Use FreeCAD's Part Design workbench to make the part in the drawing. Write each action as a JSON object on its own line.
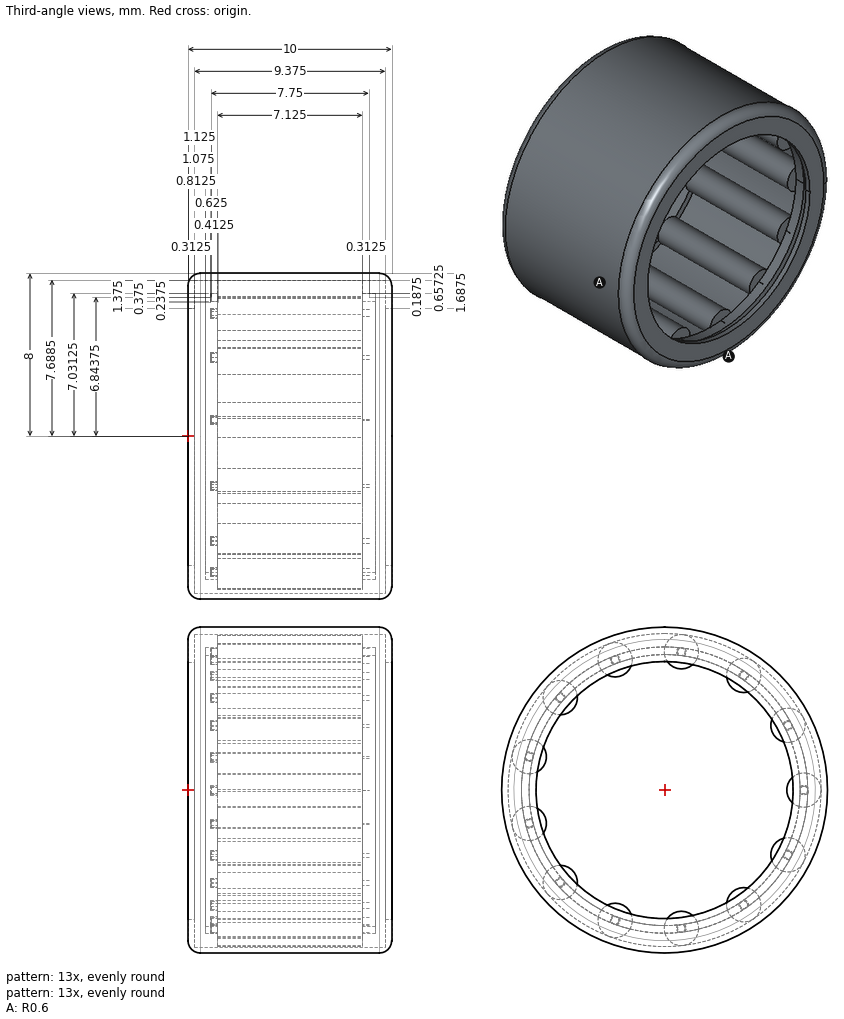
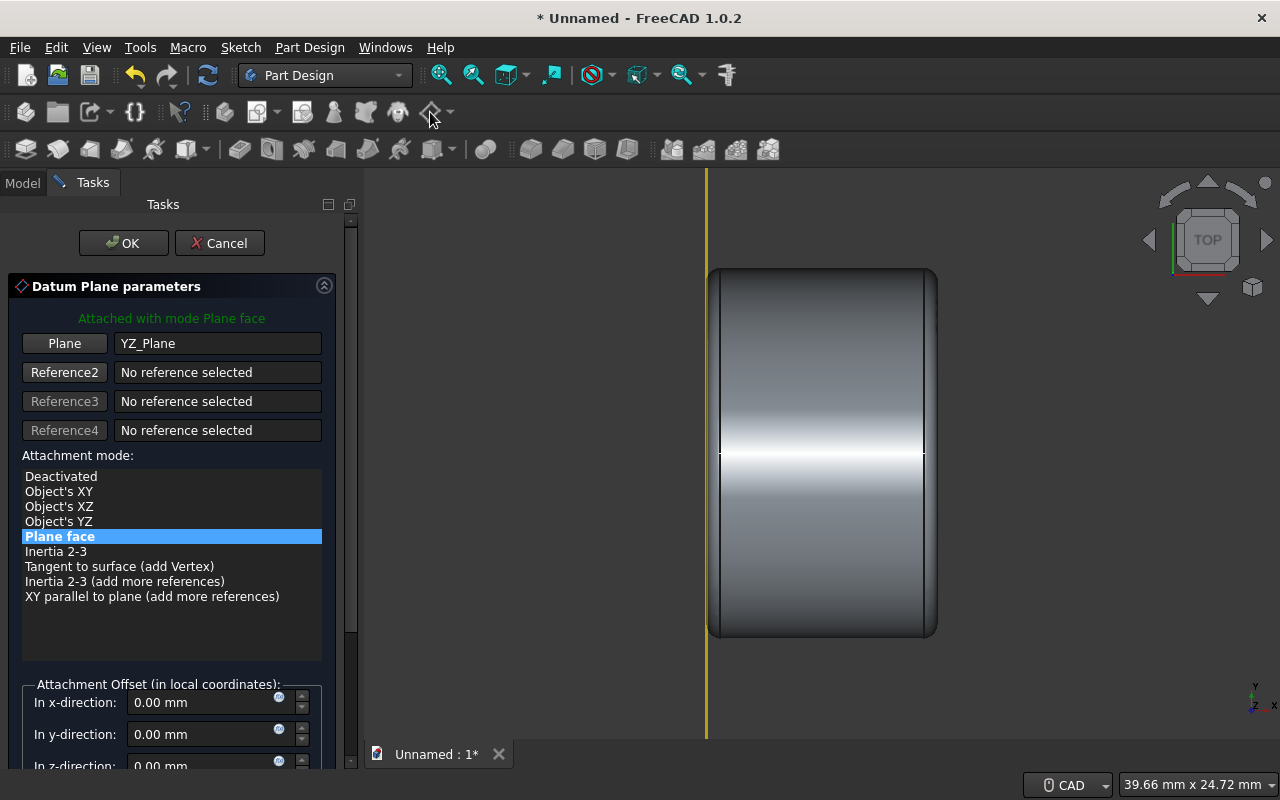
{"action": "scroll", "coordinate": [351, 491], "scroll_direction": "down", "scroll_amount": 2}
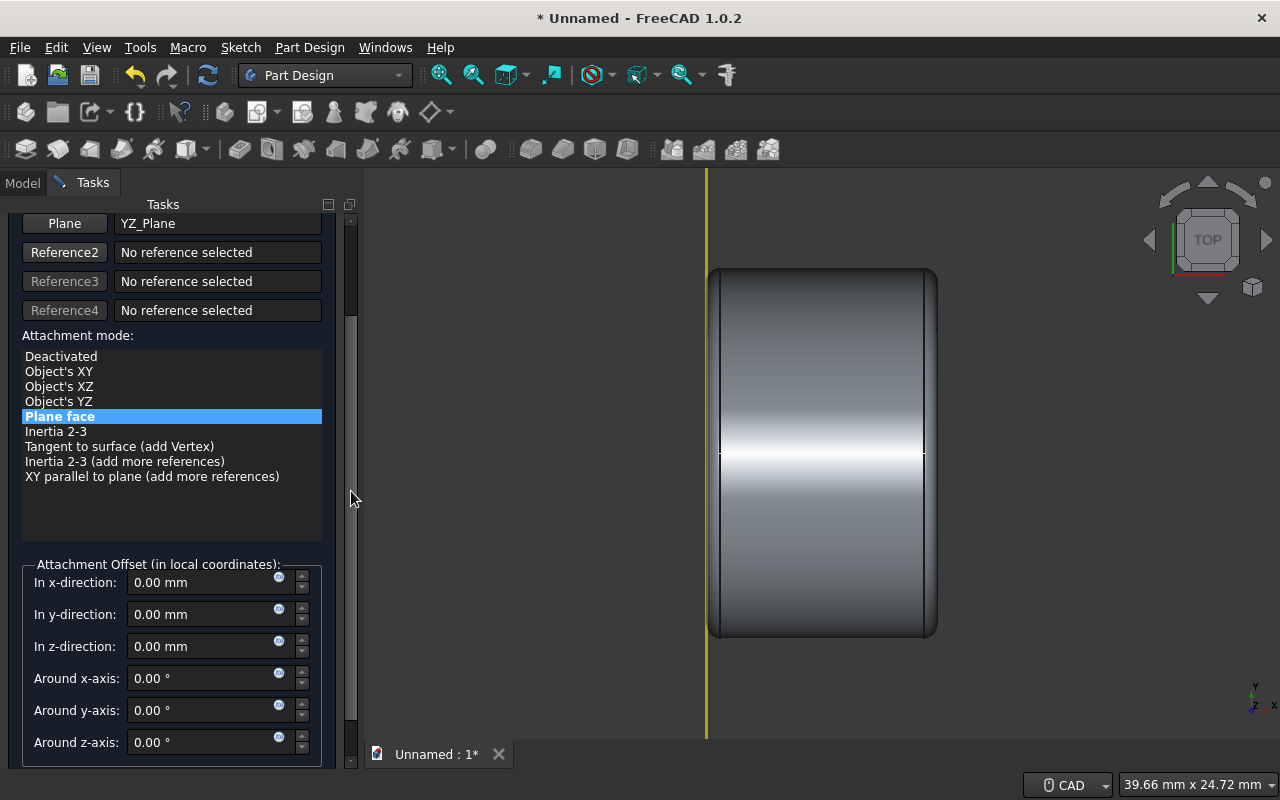
{"action": "triple_click", "coordinate": [210, 646]}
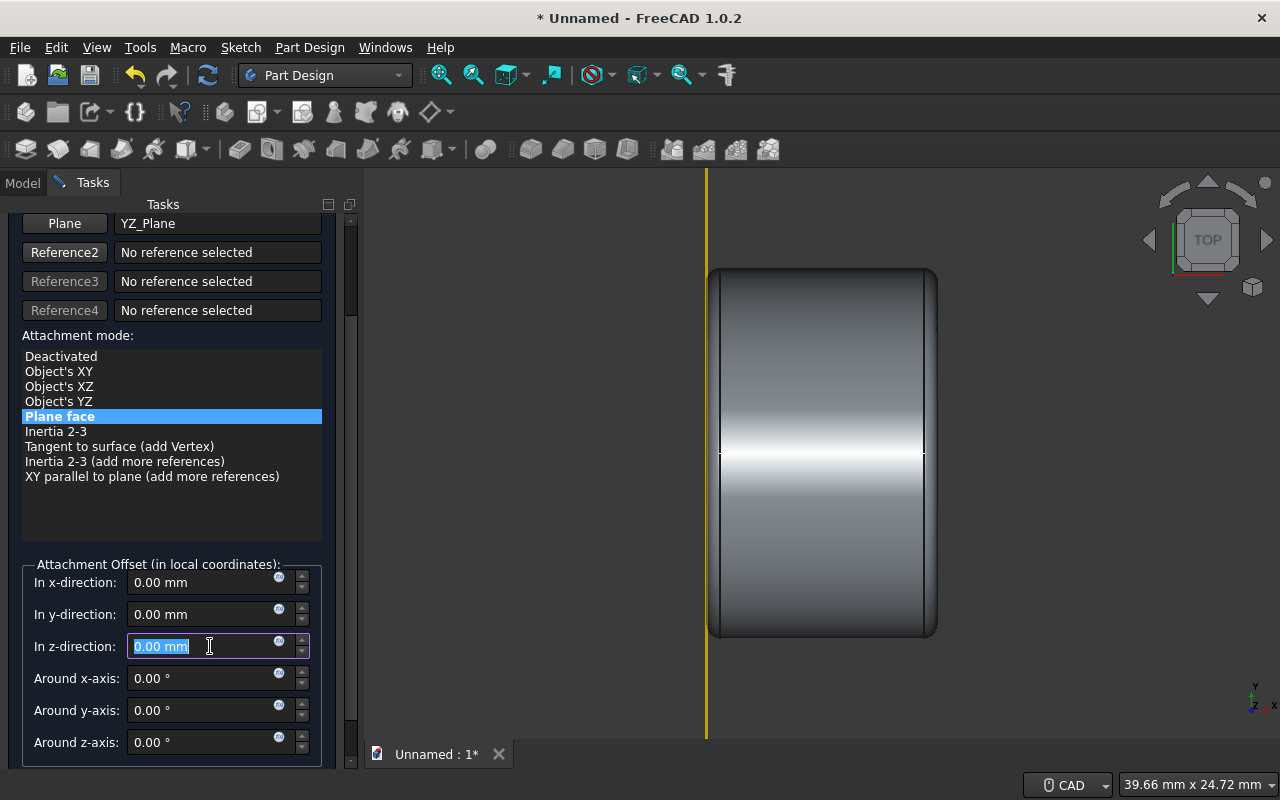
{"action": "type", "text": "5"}
{"action": "key", "text": "Tab"}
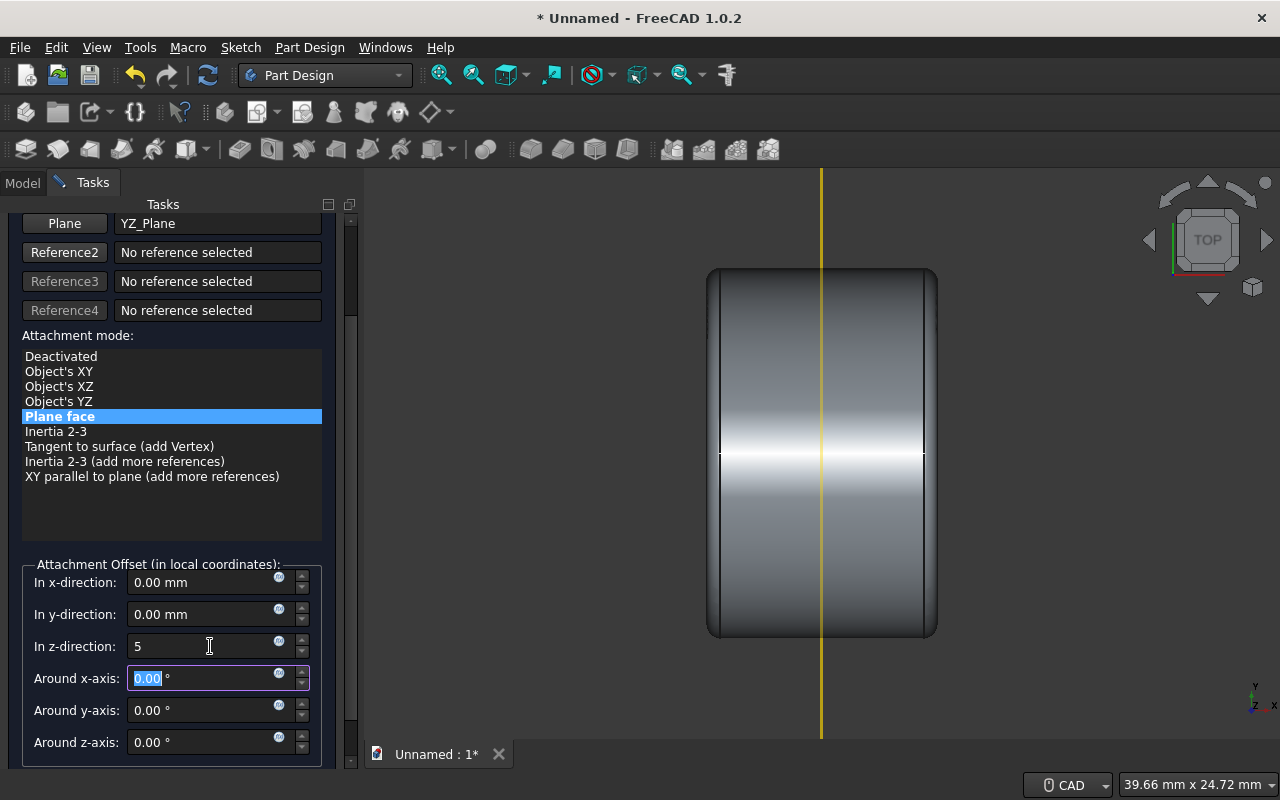
{"action": "scroll", "coordinate": [351, 491], "scroll_direction": "up", "scroll_amount": 3}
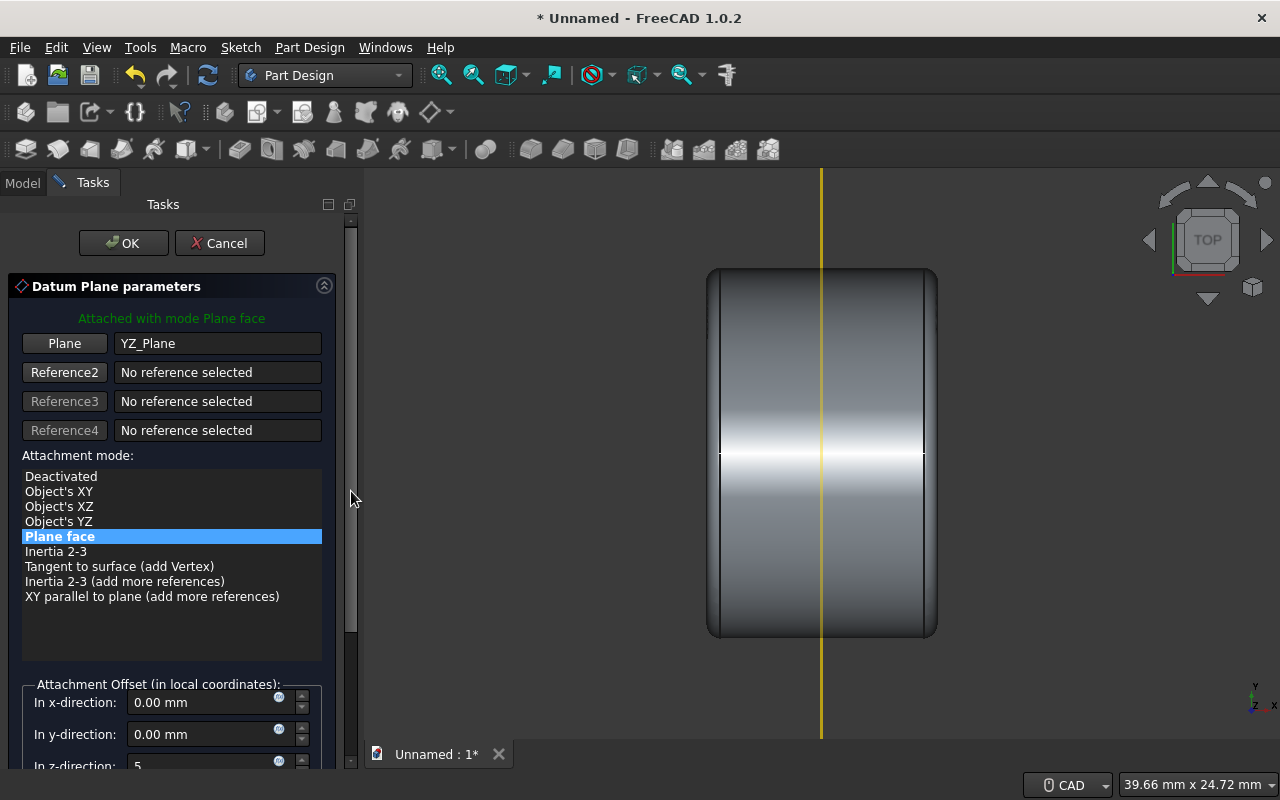
{"action": "left_click", "coordinate": [124, 243]}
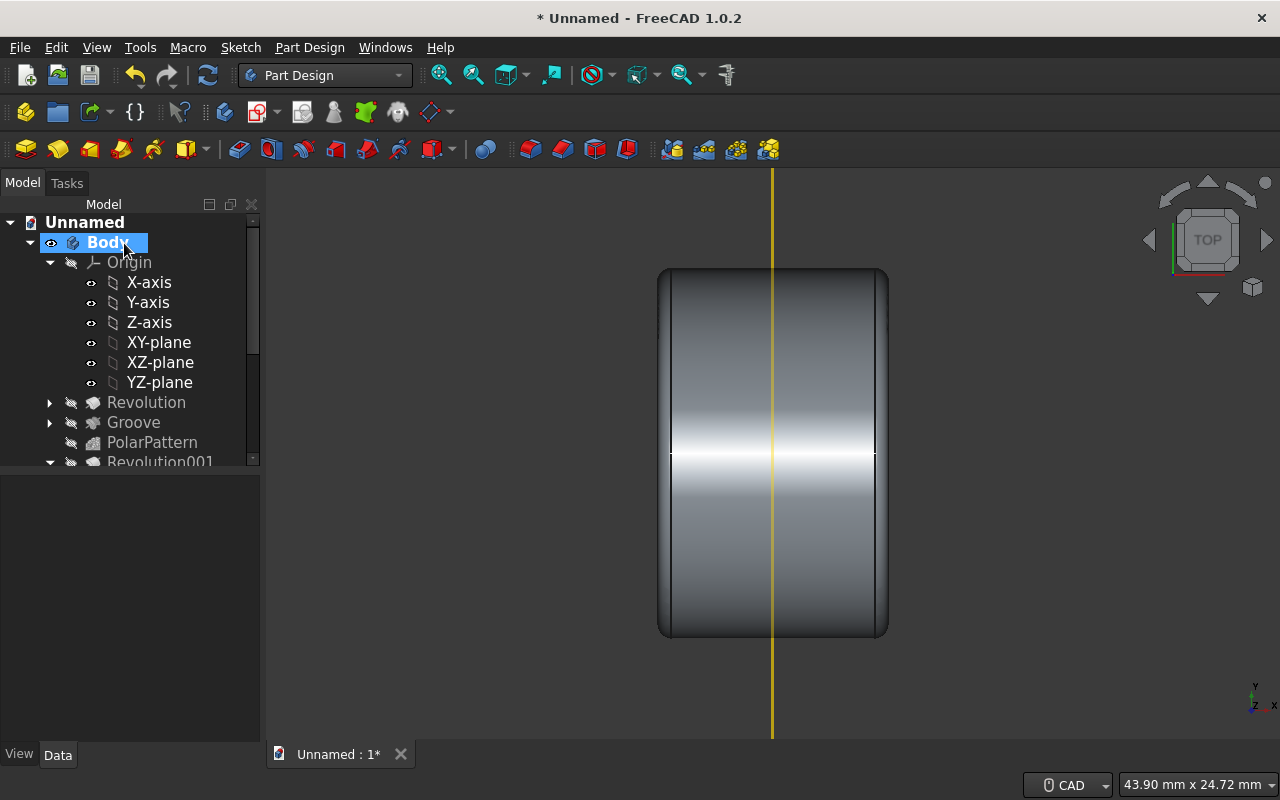
{"action": "left_click", "coordinate": [116, 463]}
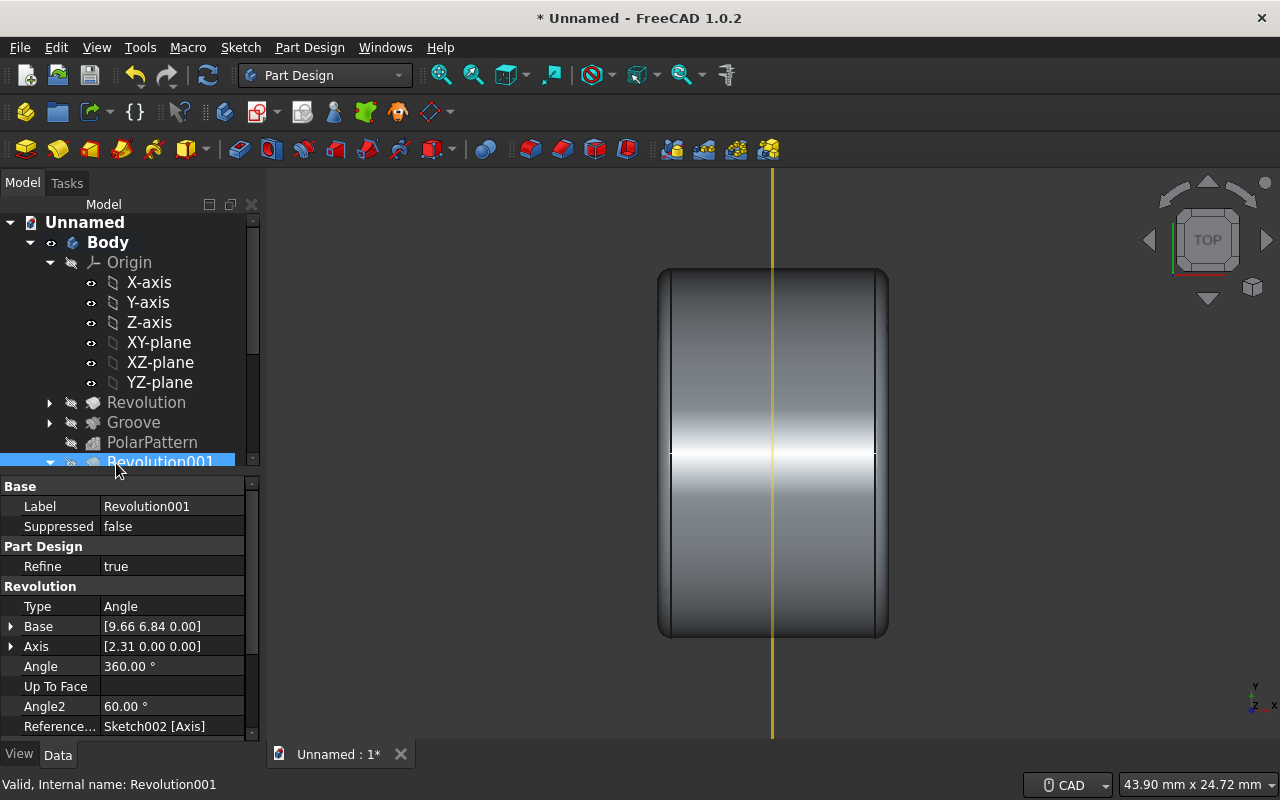
{"action": "left_click", "coordinate": [672, 150]}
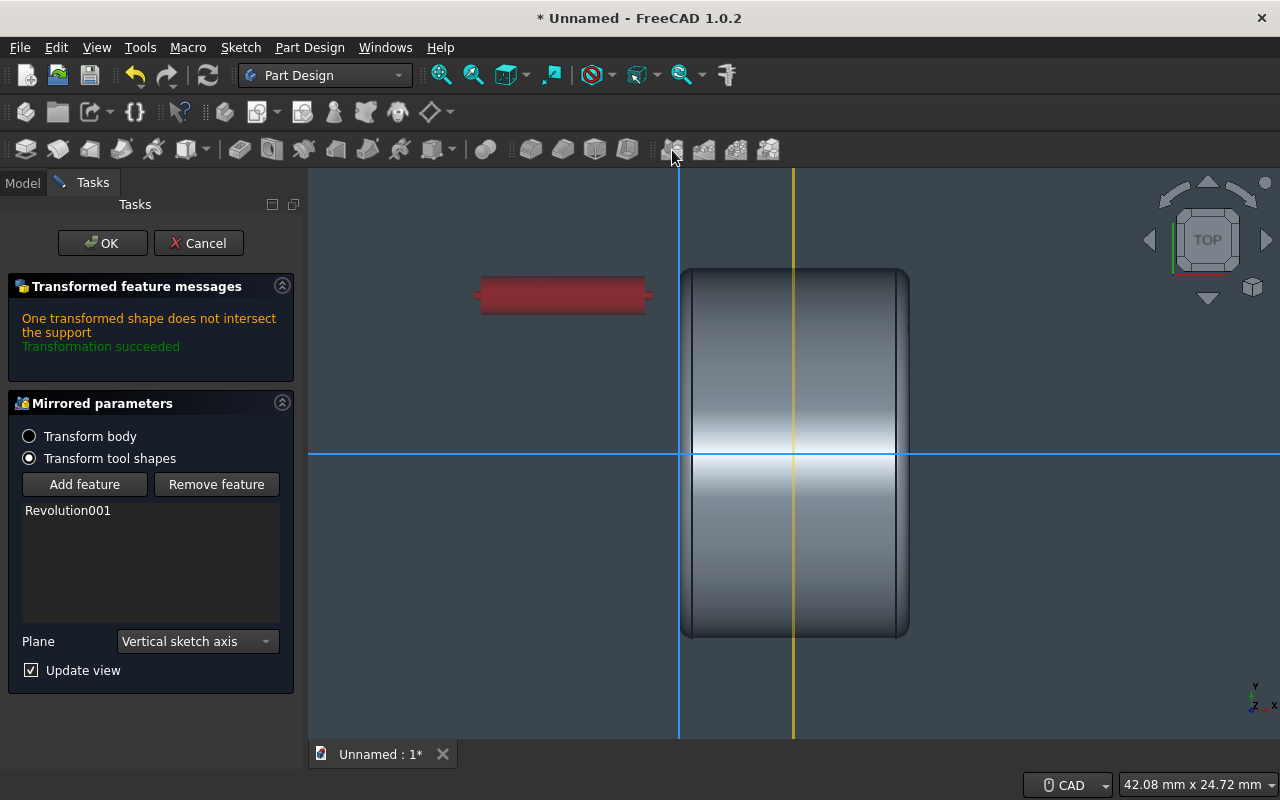
{"action": "left_click", "coordinate": [198, 642]}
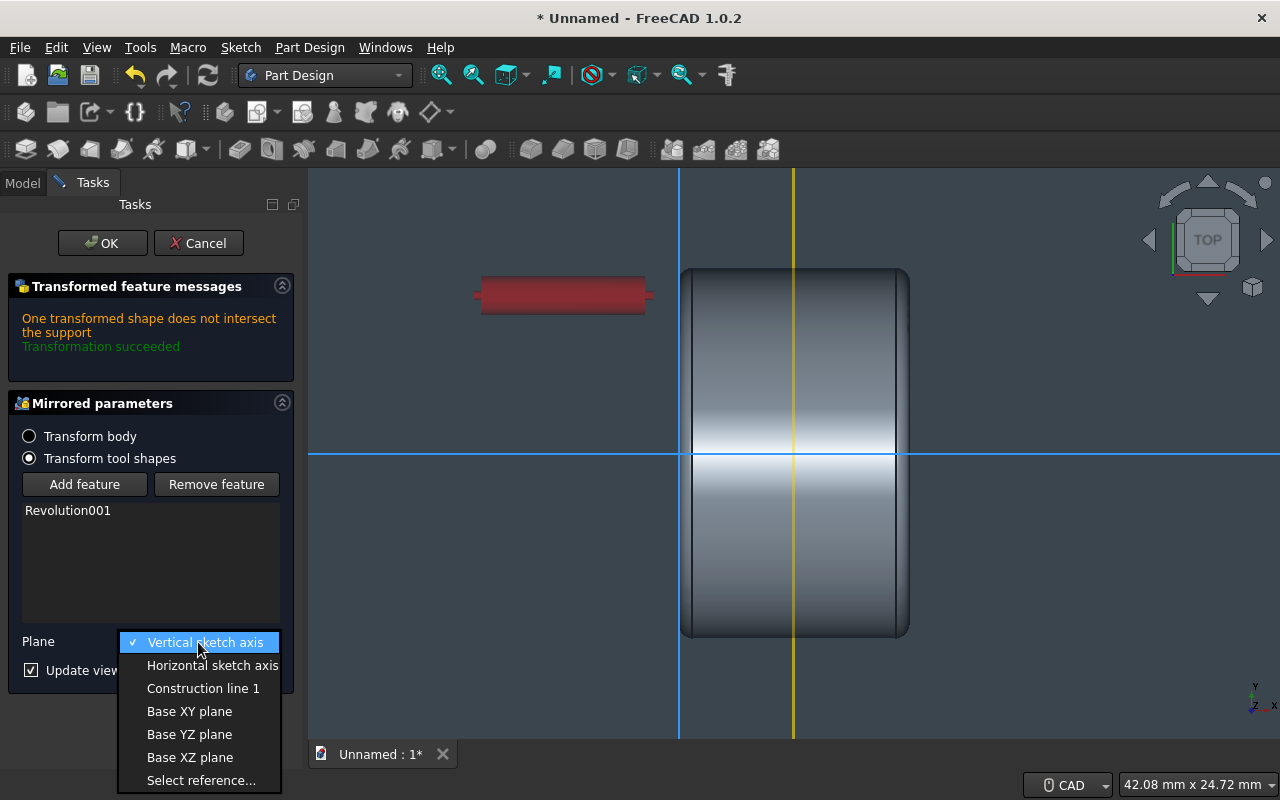
{"action": "left_click", "coordinate": [198, 780]}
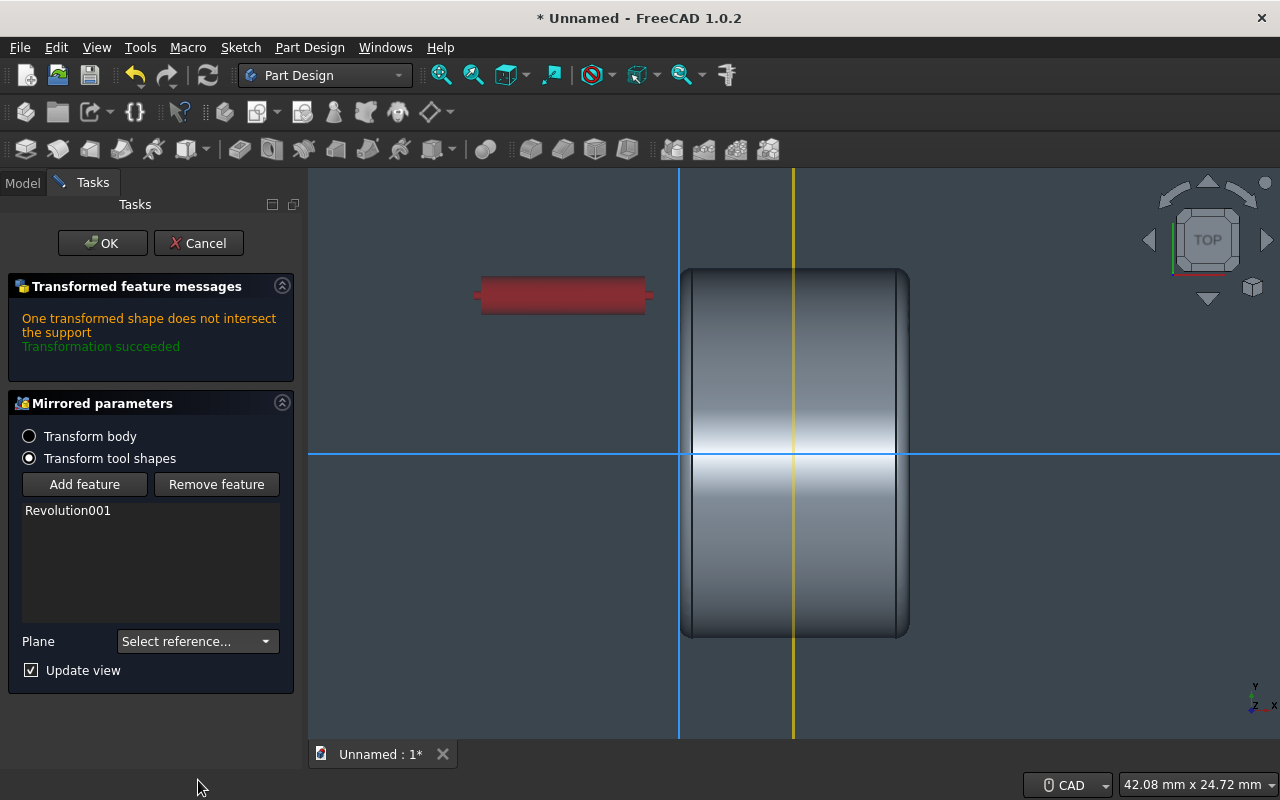
{"action": "left_click", "coordinate": [23, 182]}